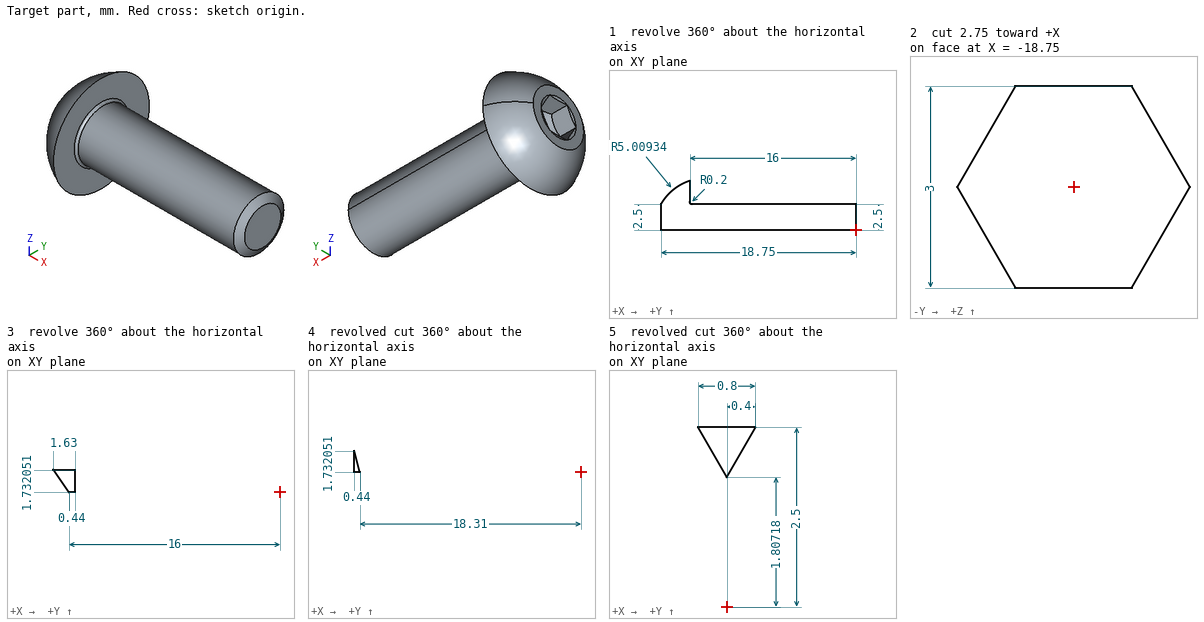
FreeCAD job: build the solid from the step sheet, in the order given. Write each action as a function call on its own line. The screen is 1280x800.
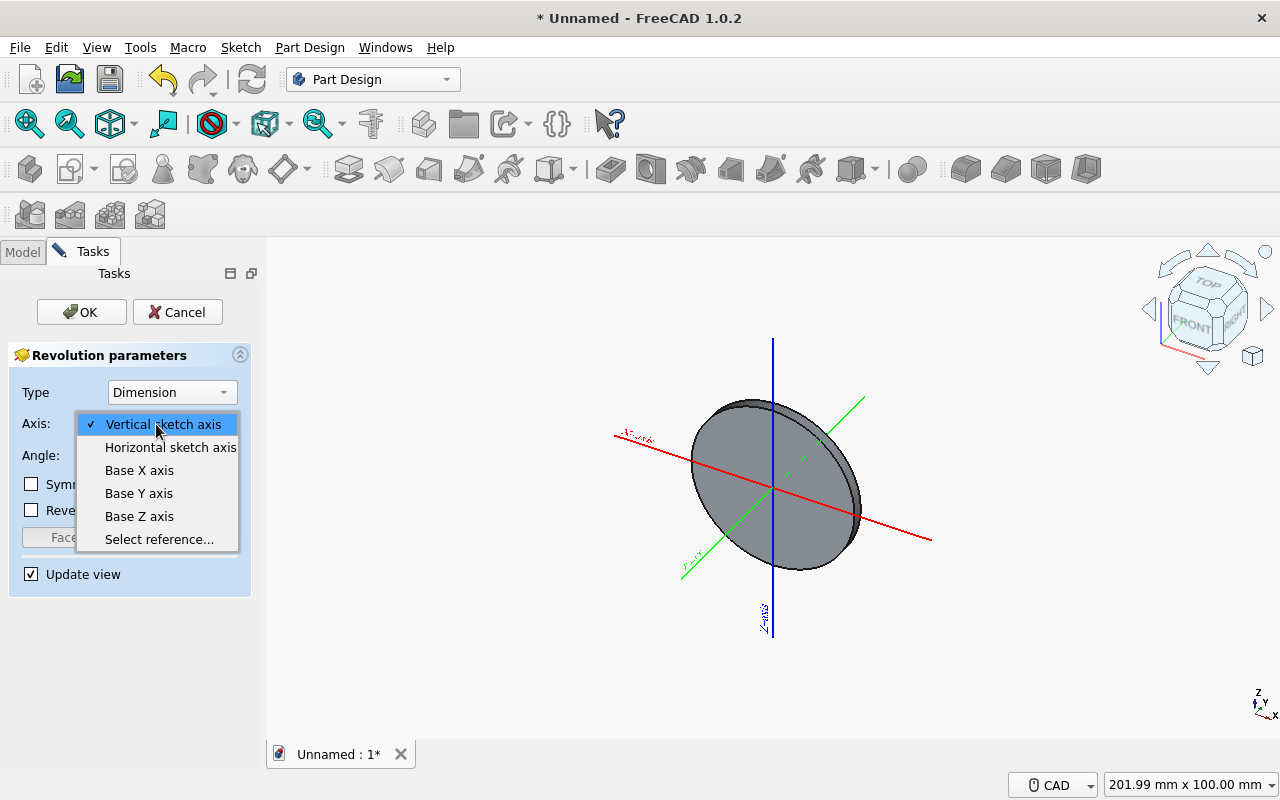
click(156, 448)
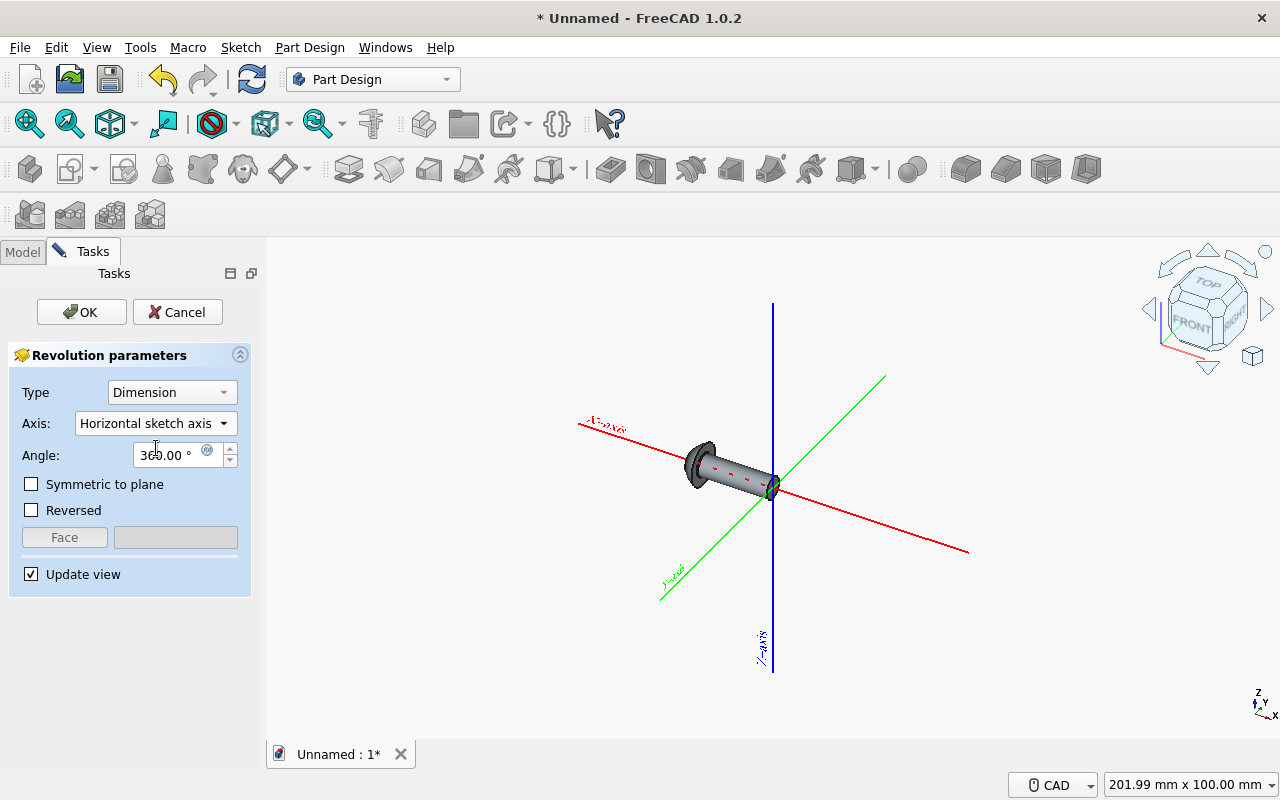
click(82, 312)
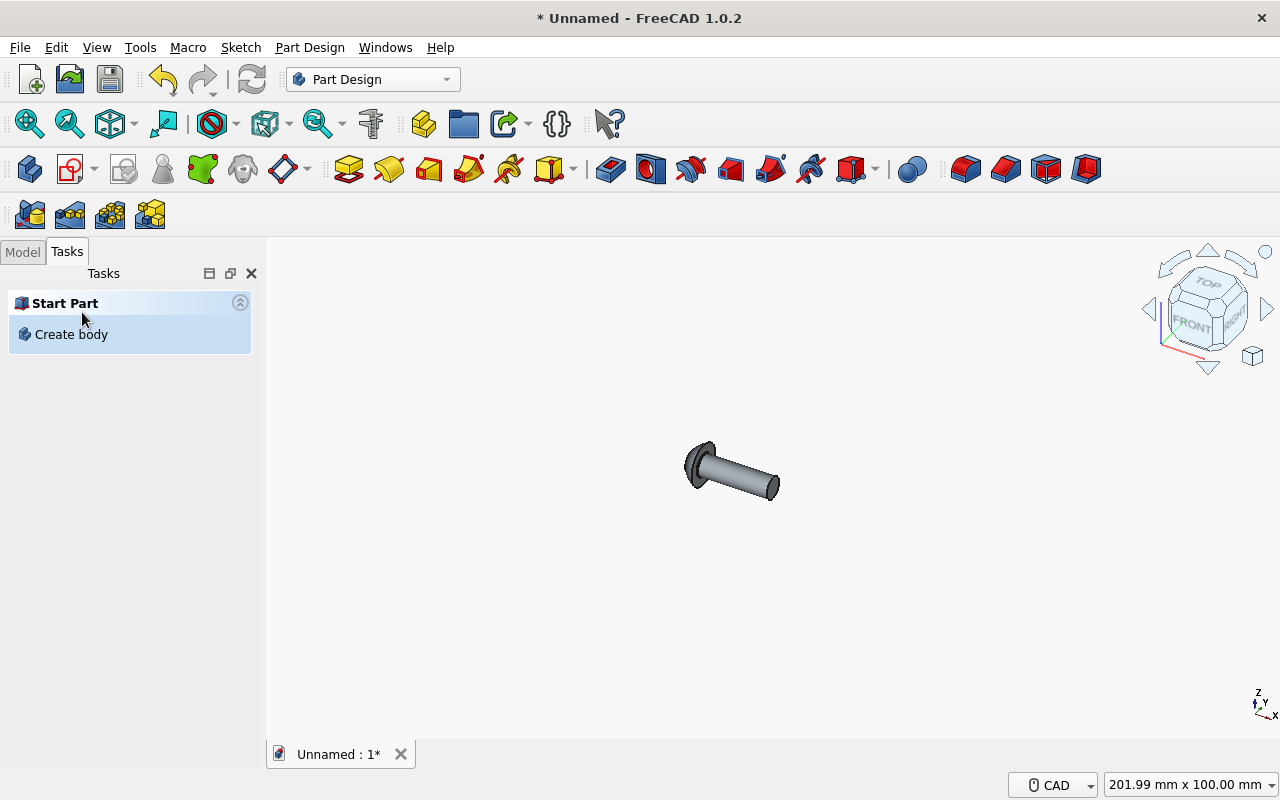
click(30, 124)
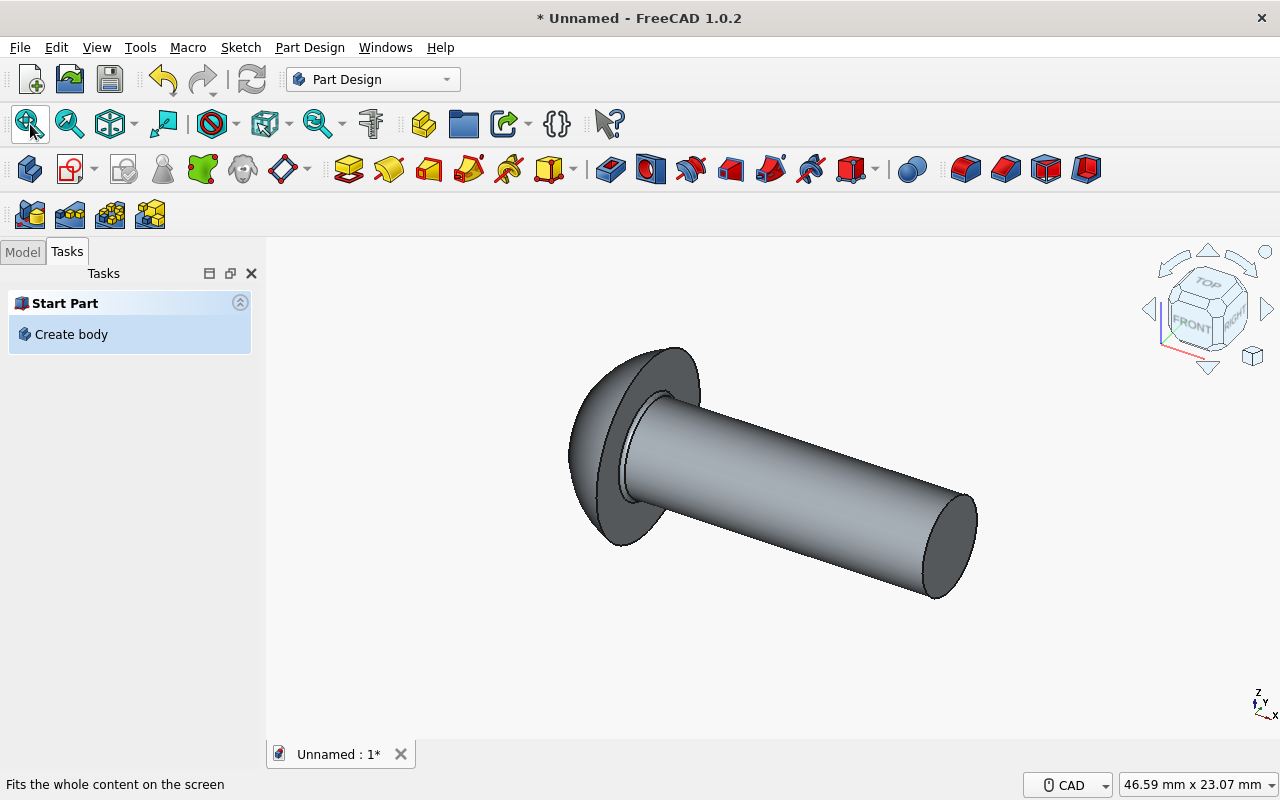
key(6)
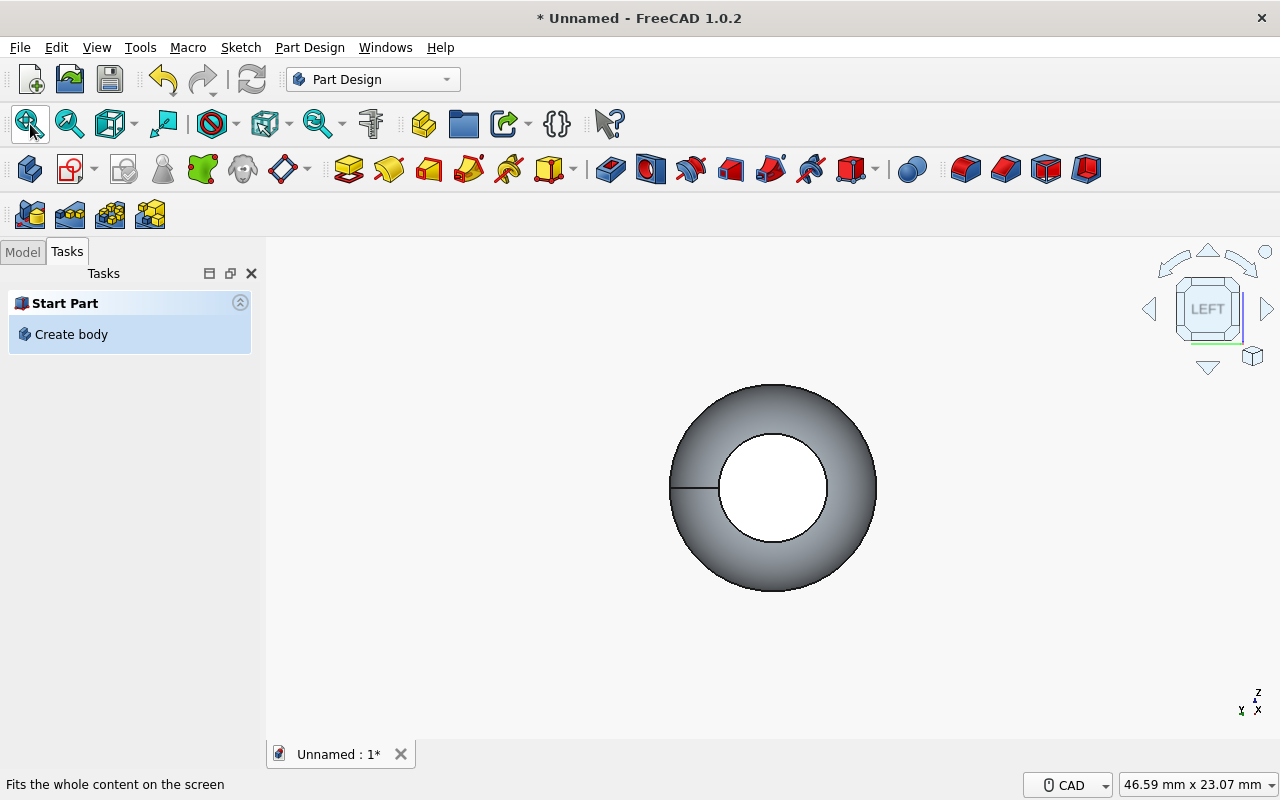
click(30, 124)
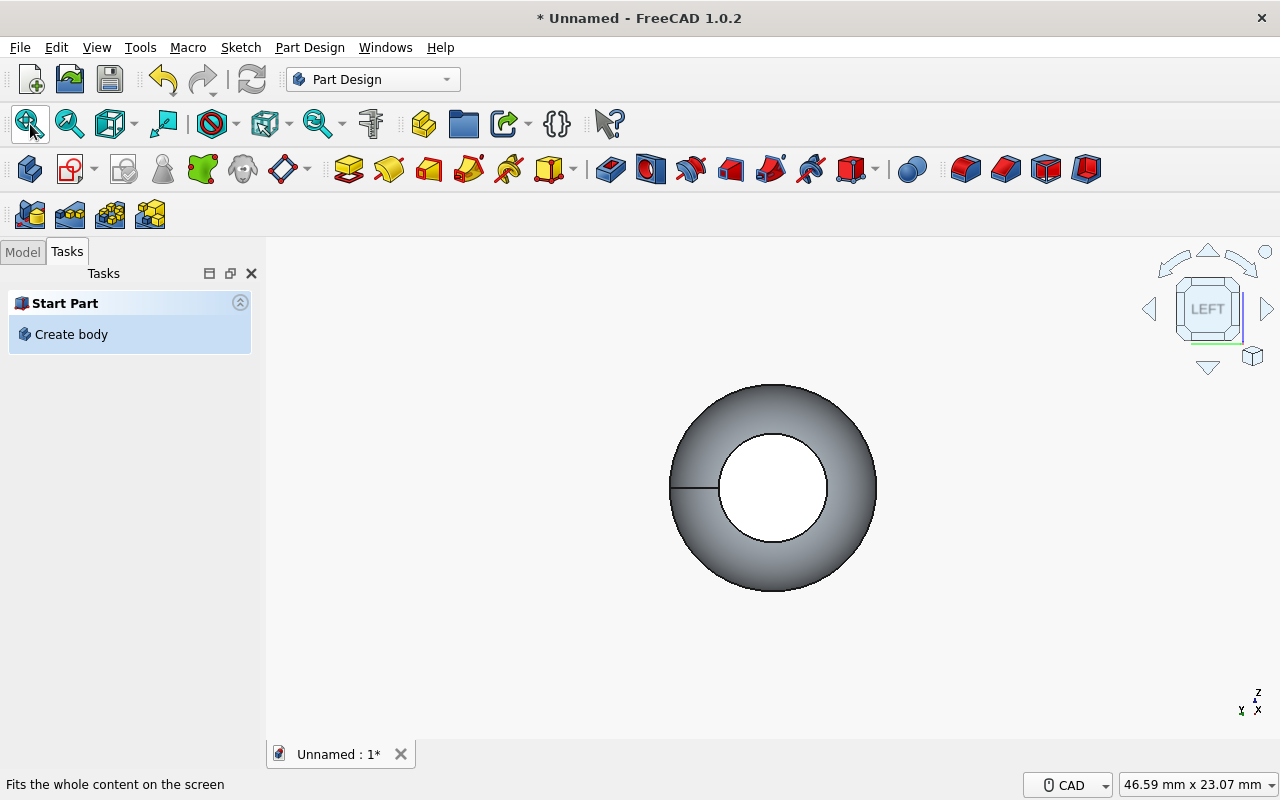
click(773, 487)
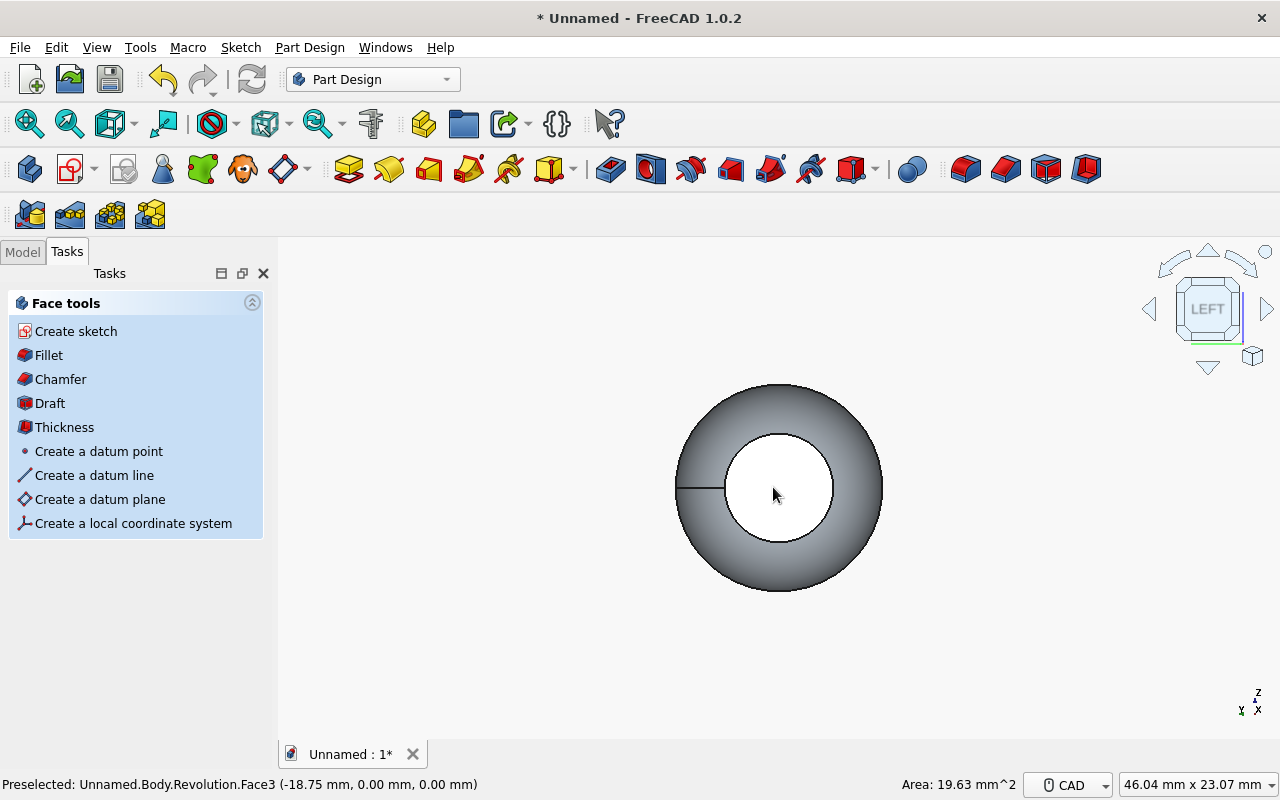
click(70, 170)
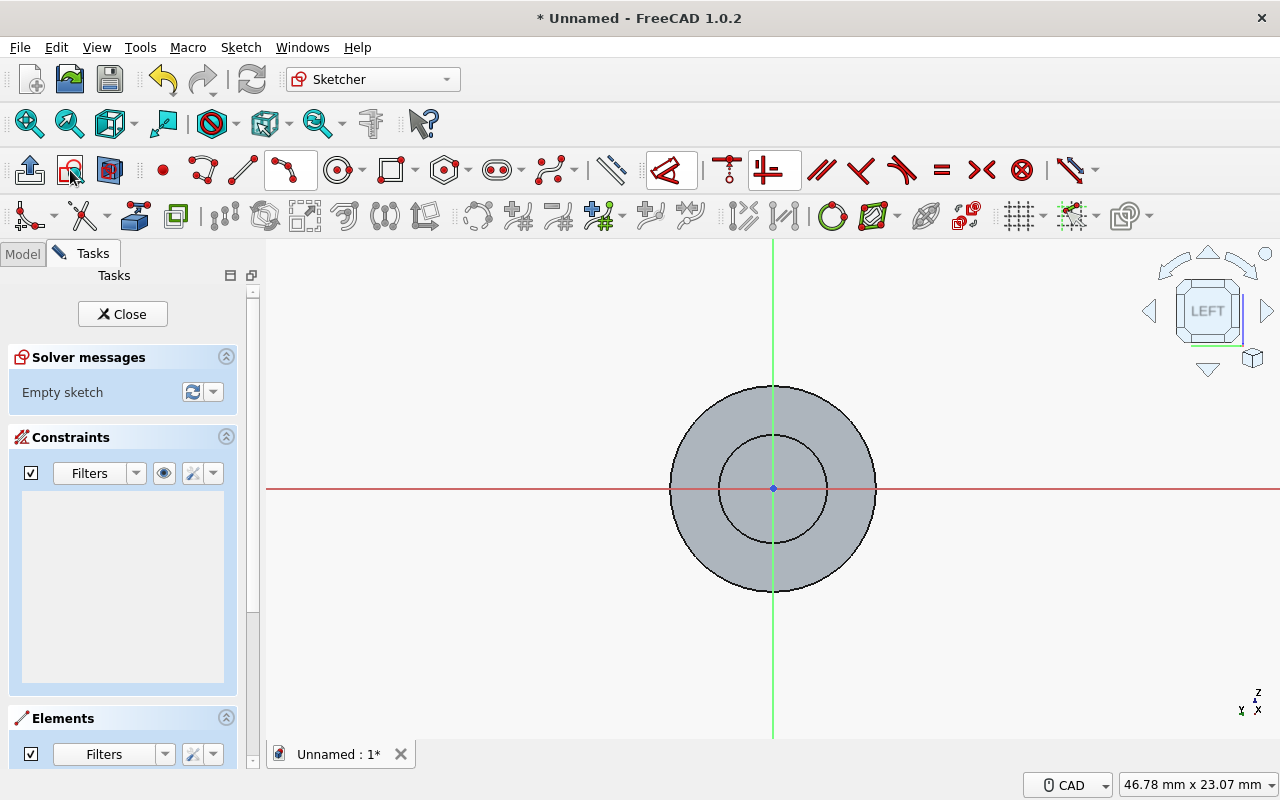
scroll(790, 489, up, 8)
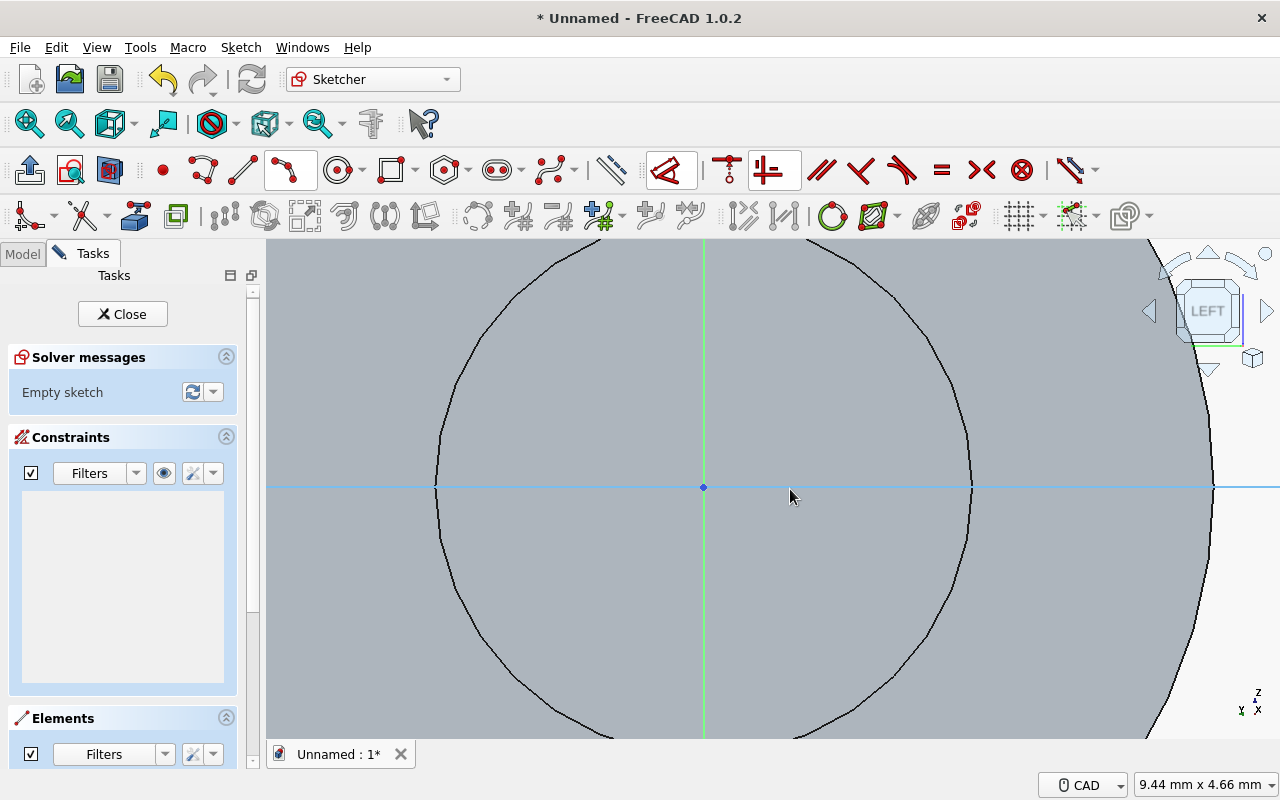
click(444, 170)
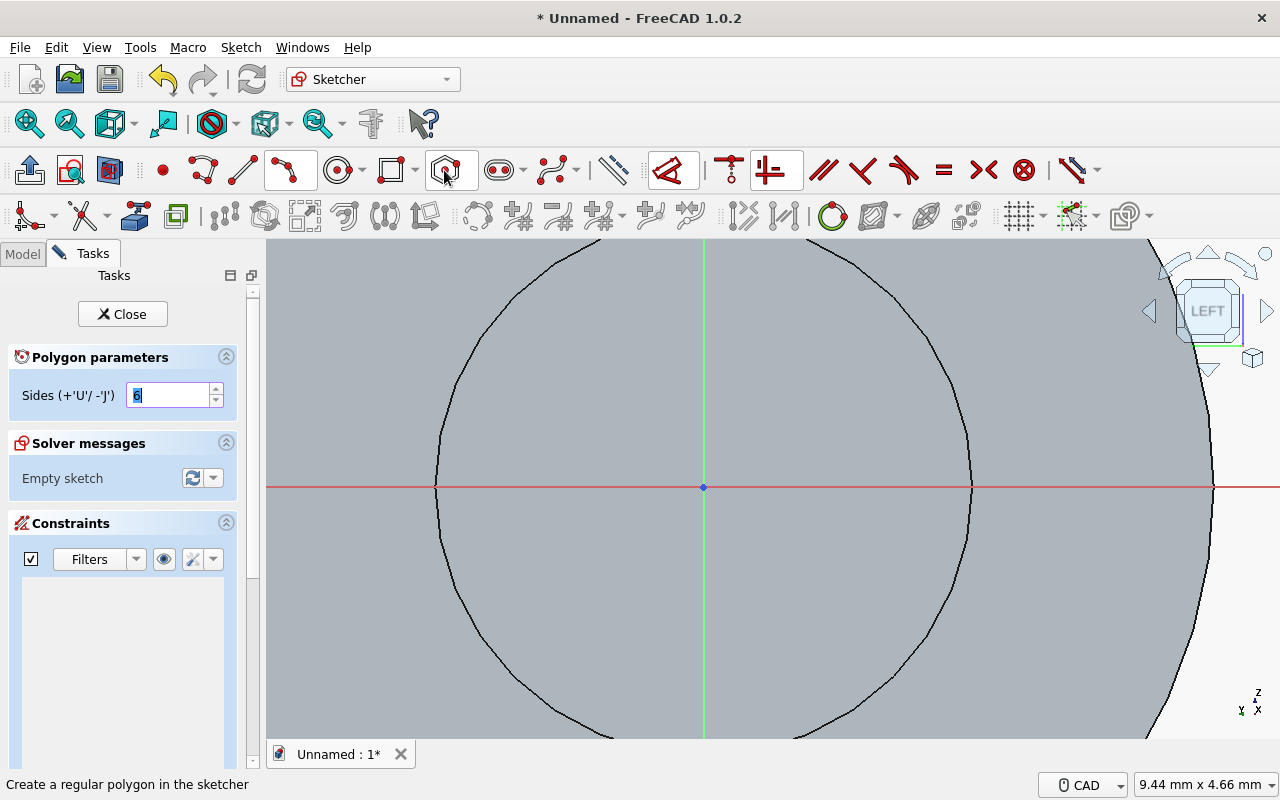
click(704, 487)